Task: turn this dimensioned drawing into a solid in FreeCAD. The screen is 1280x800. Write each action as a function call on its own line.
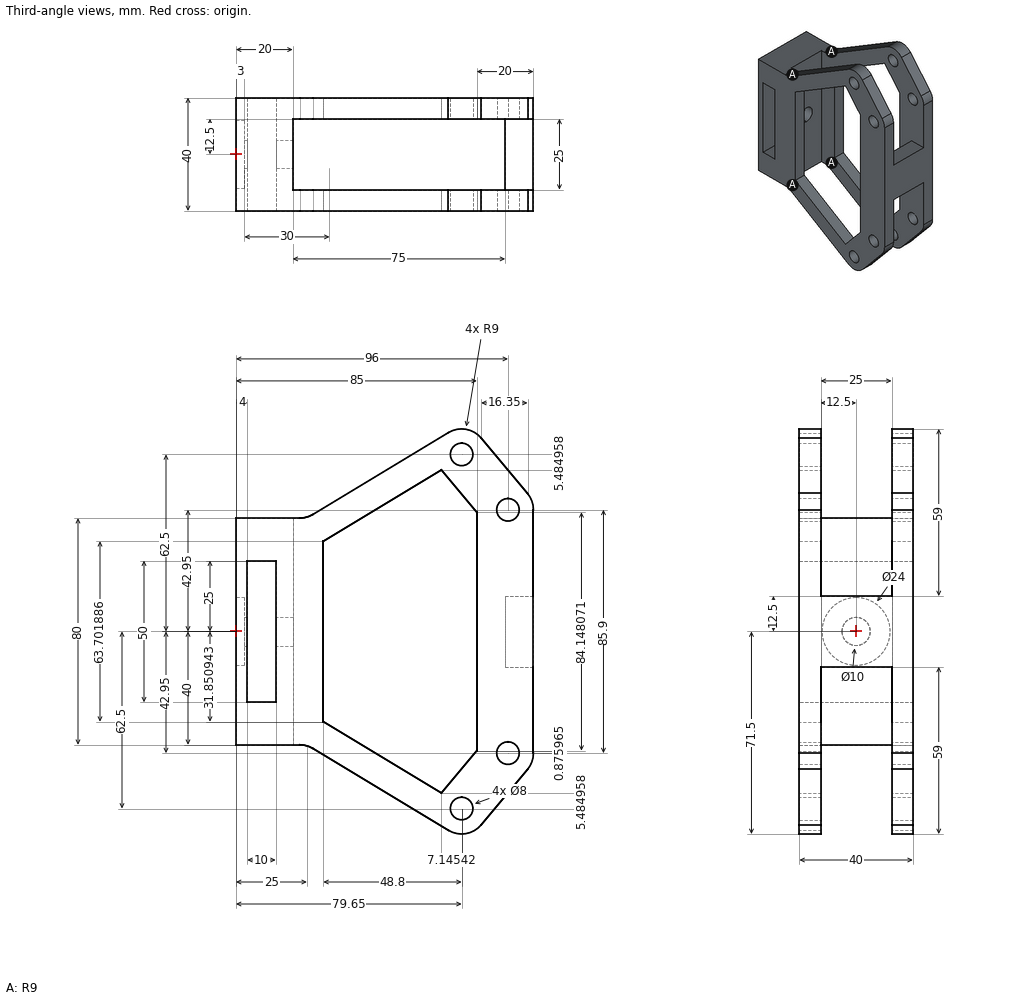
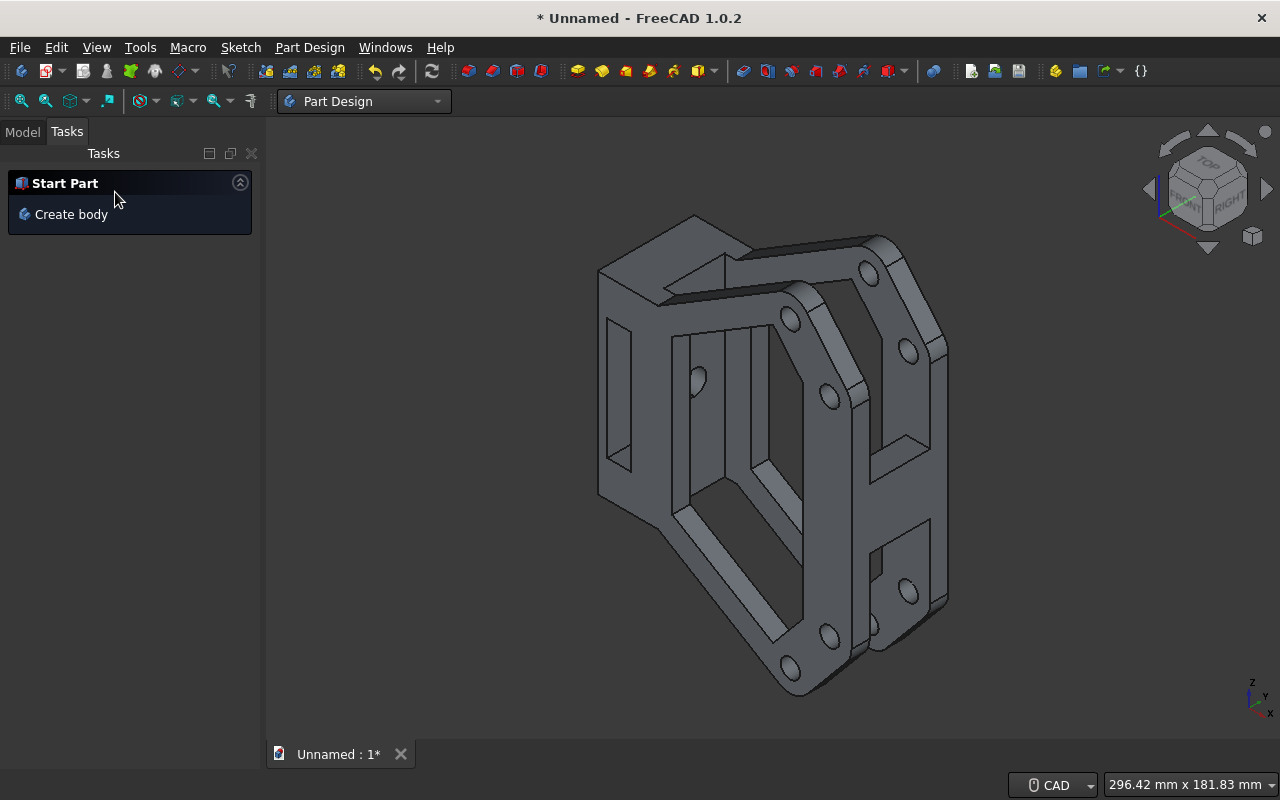
key(2)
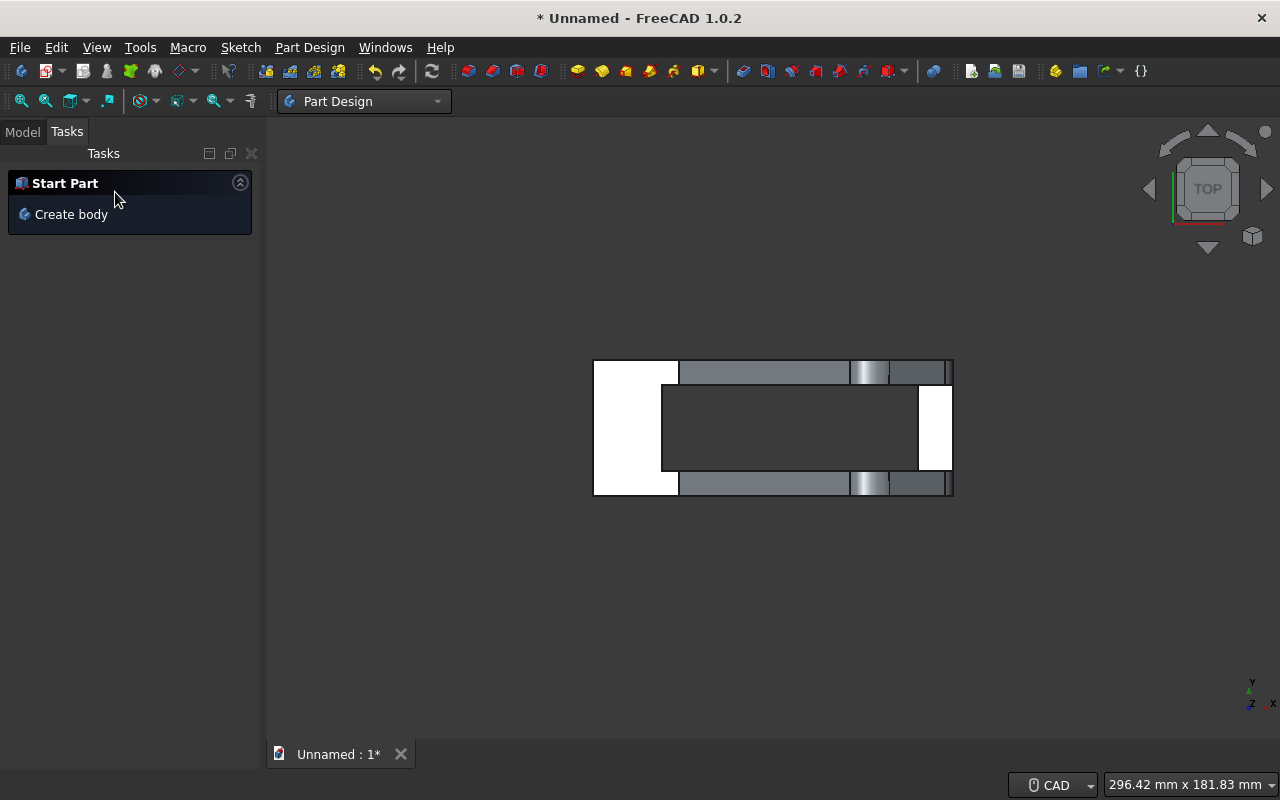
key(v)
key(f)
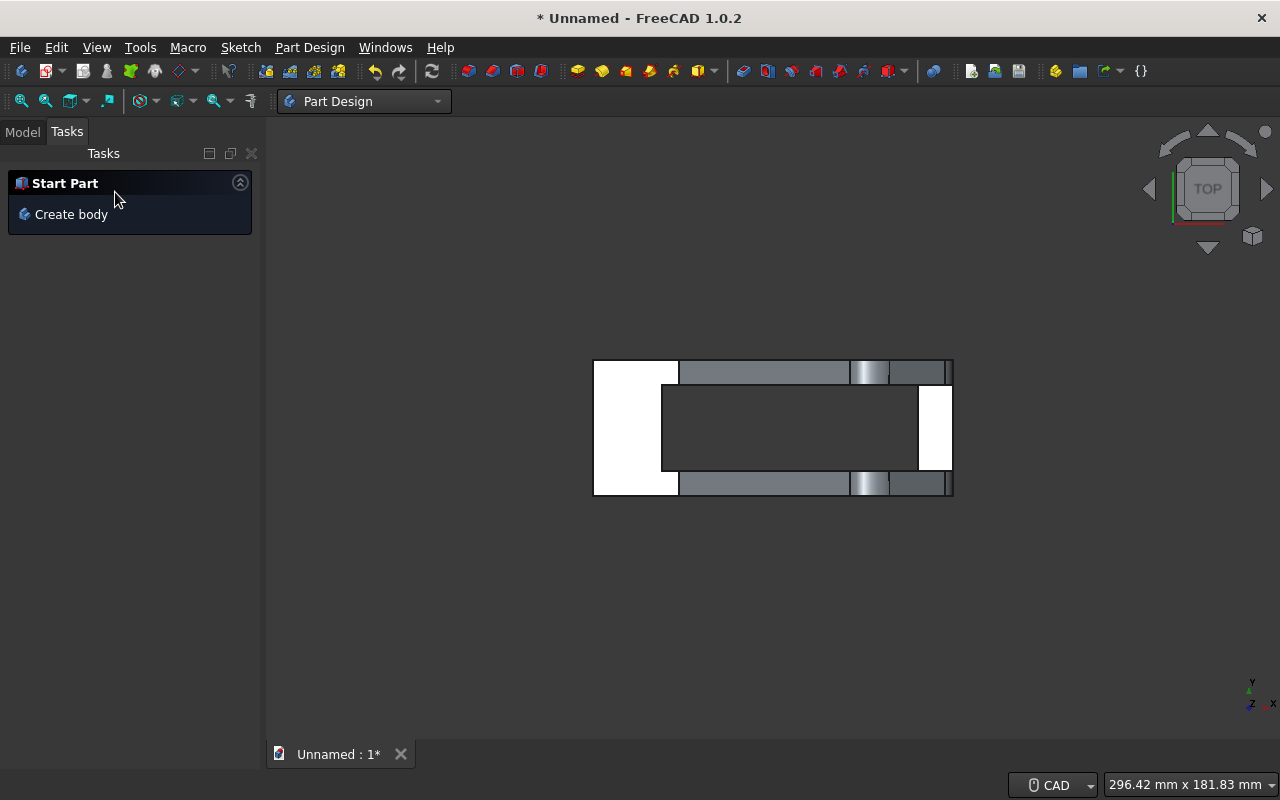
key(1)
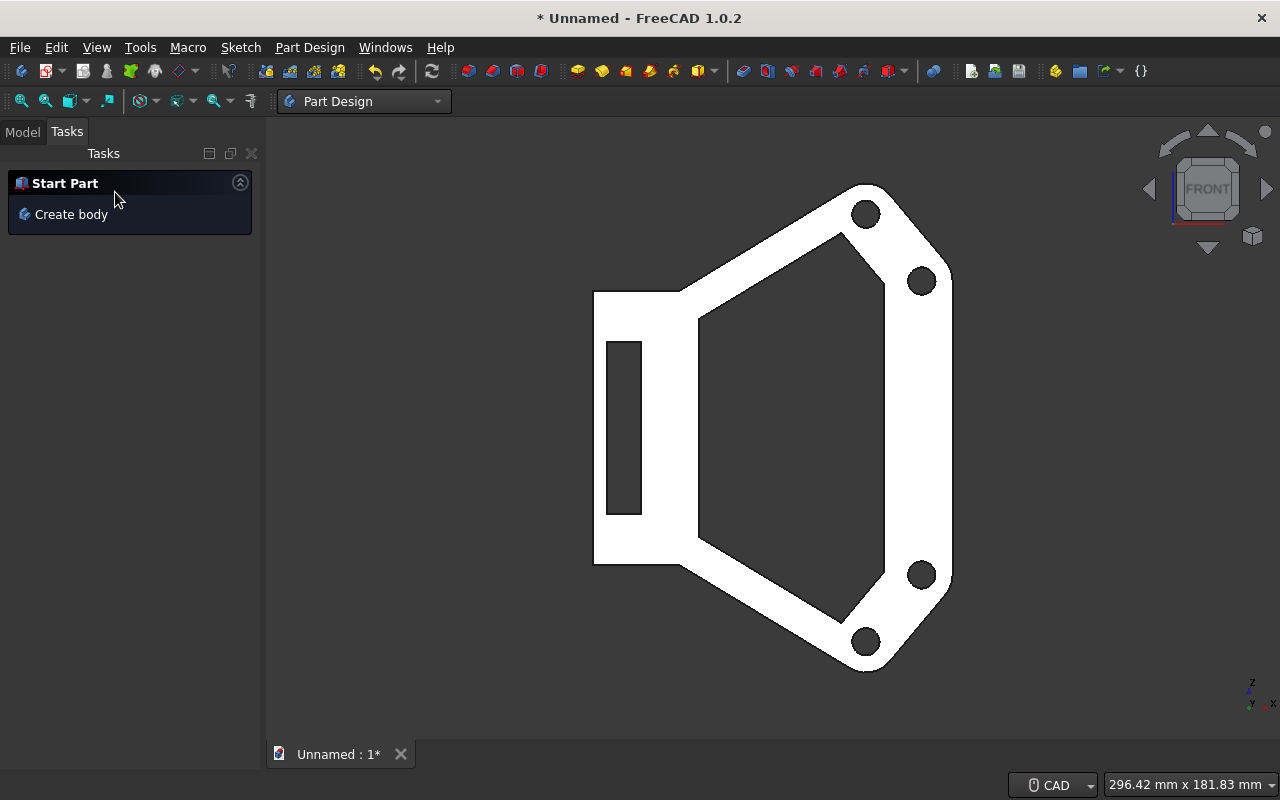
key(3)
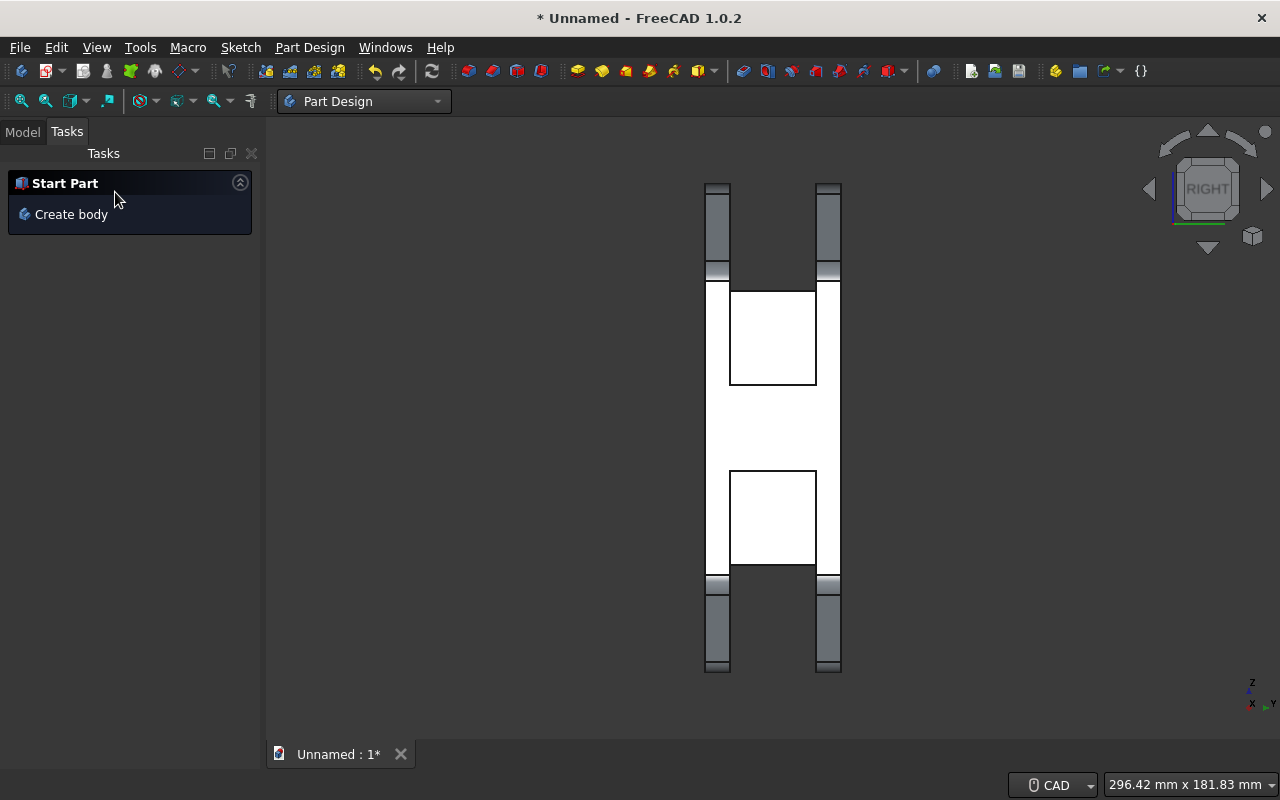
key(5)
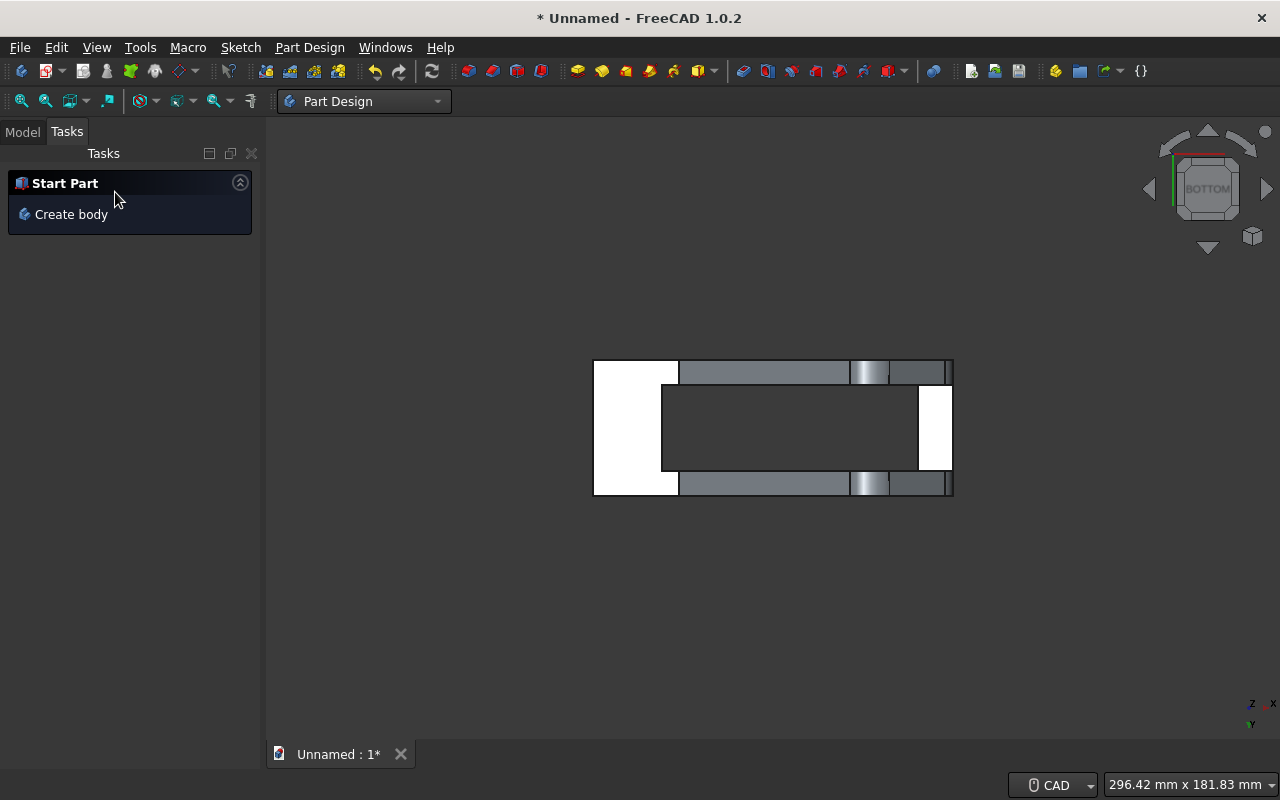
click(22, 102)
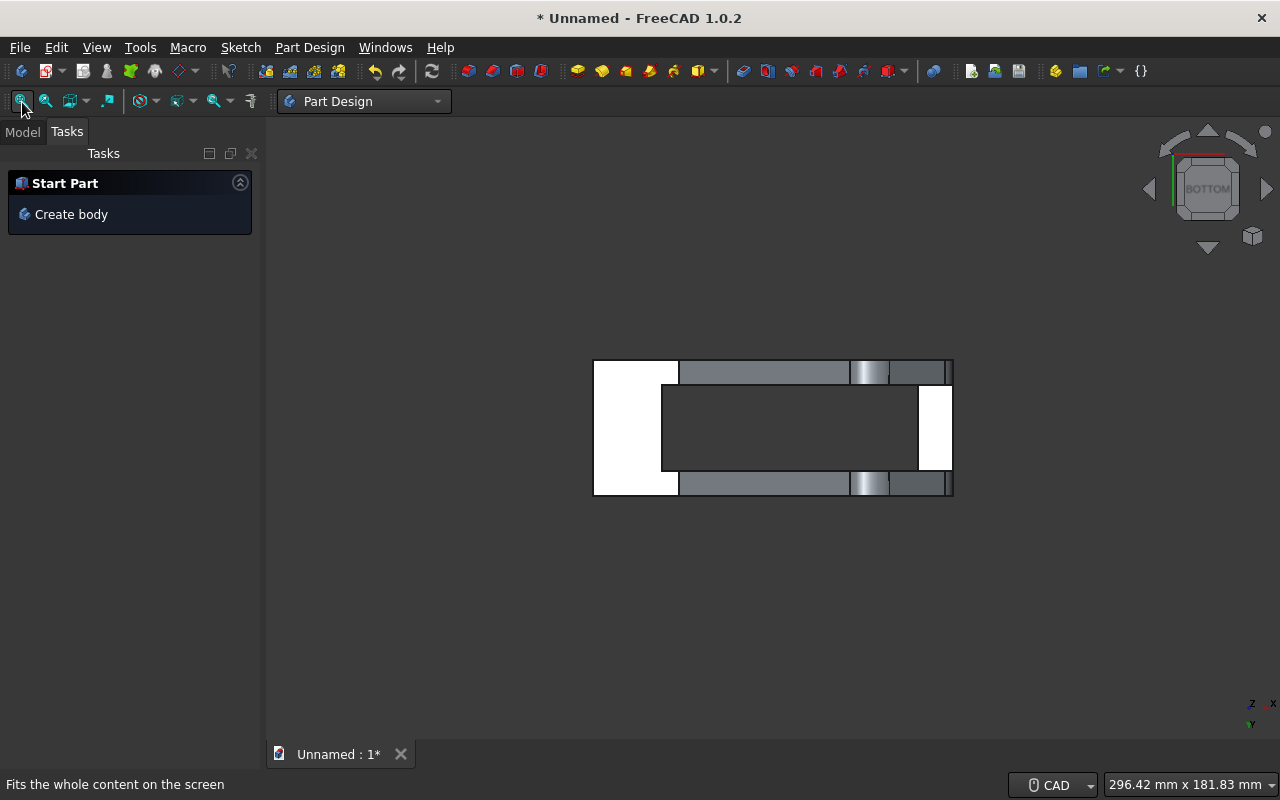
key(4)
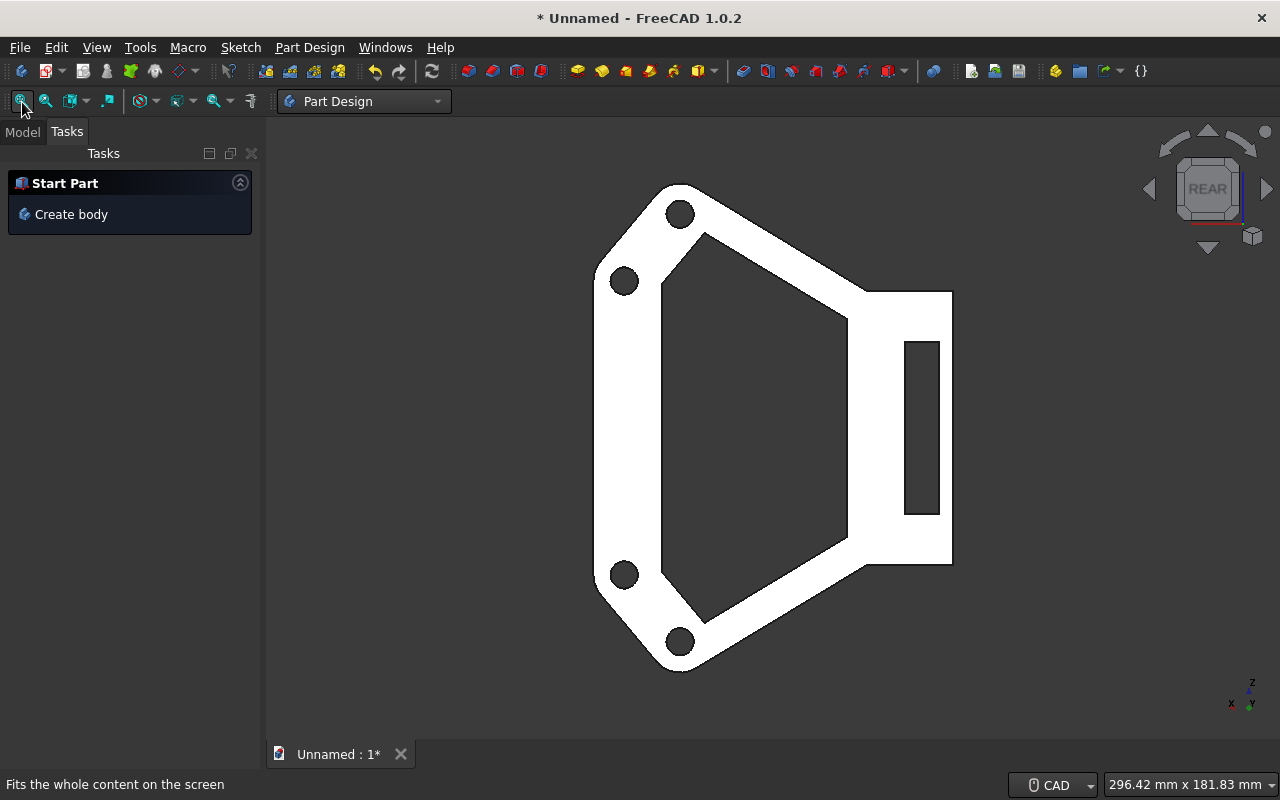
key(6)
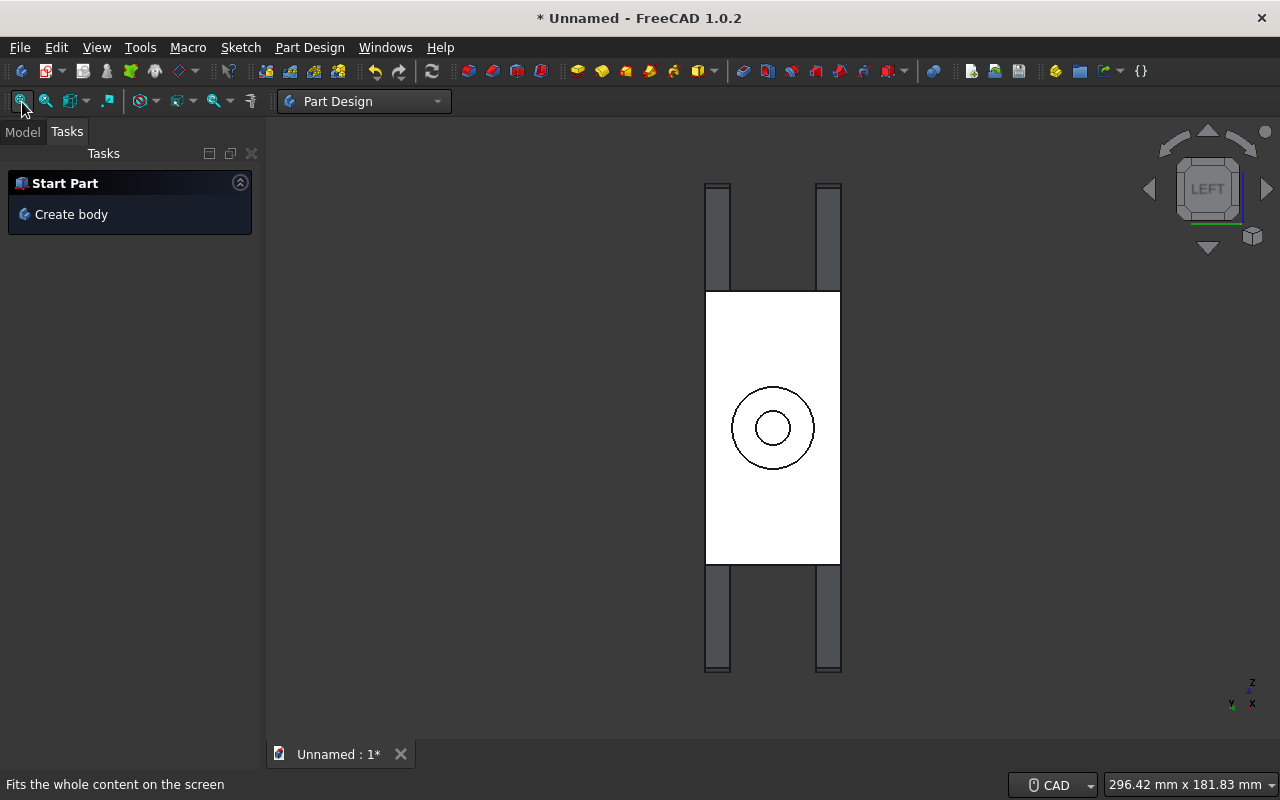
key(v)
key(3)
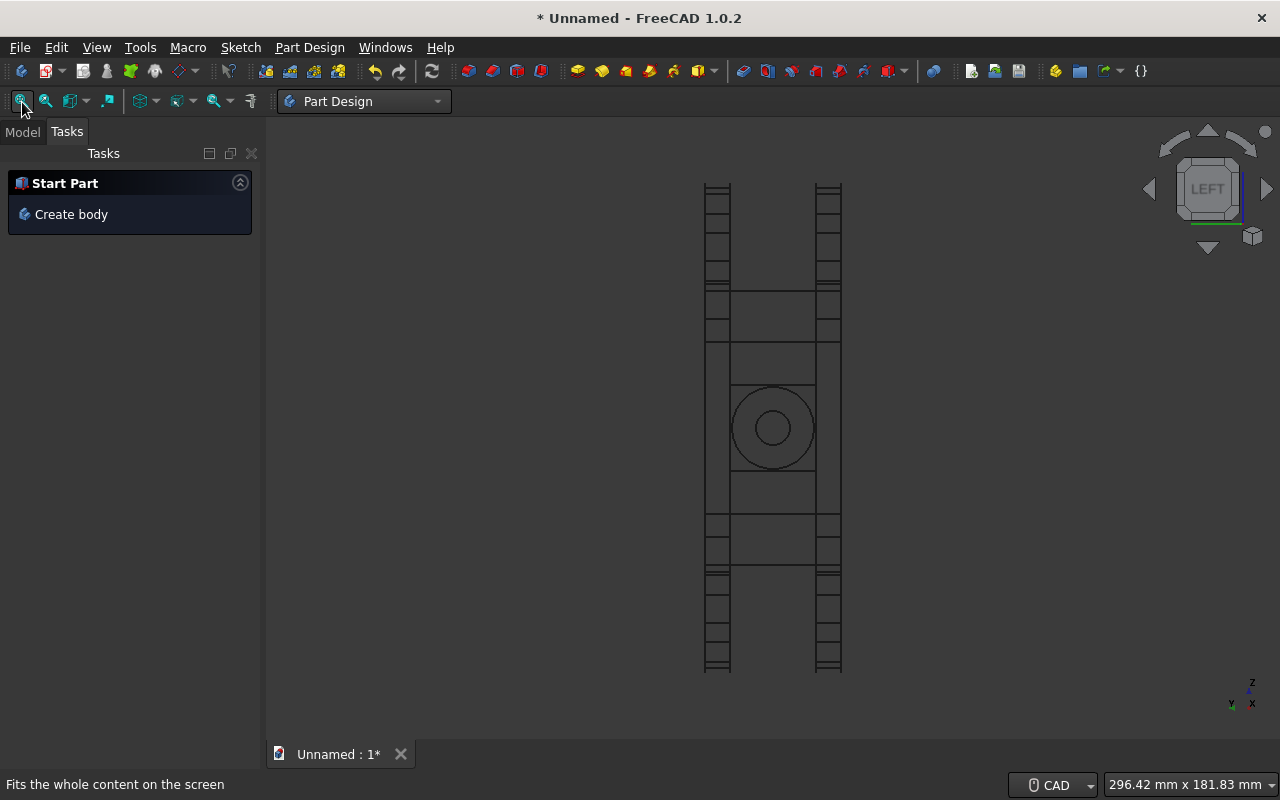
key(0)